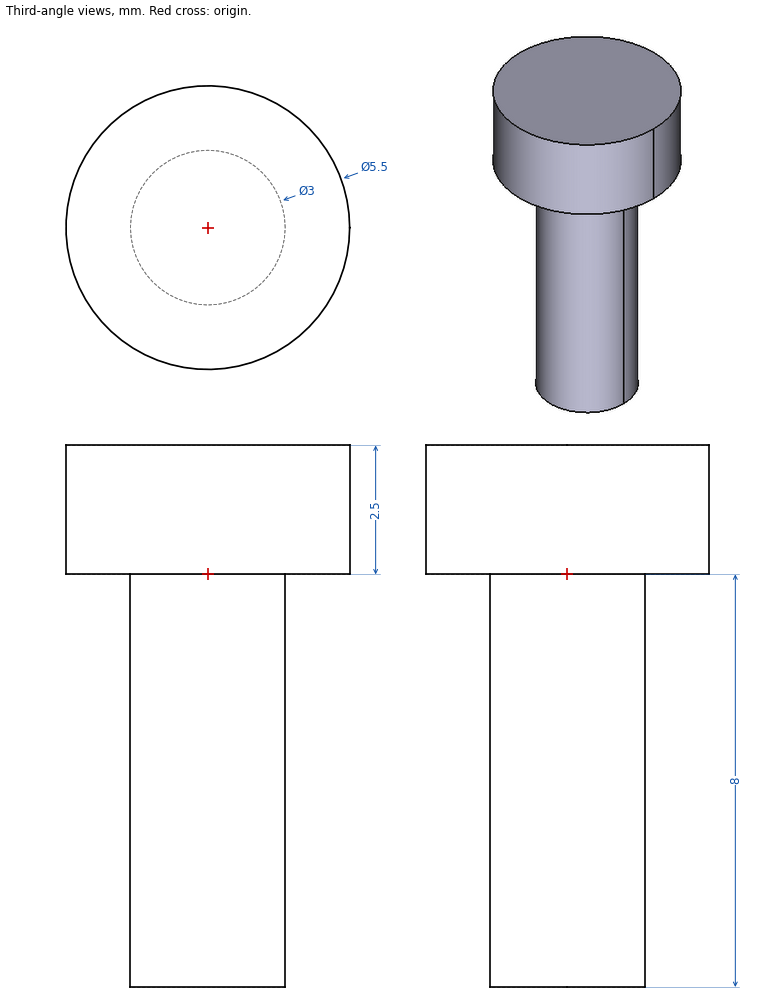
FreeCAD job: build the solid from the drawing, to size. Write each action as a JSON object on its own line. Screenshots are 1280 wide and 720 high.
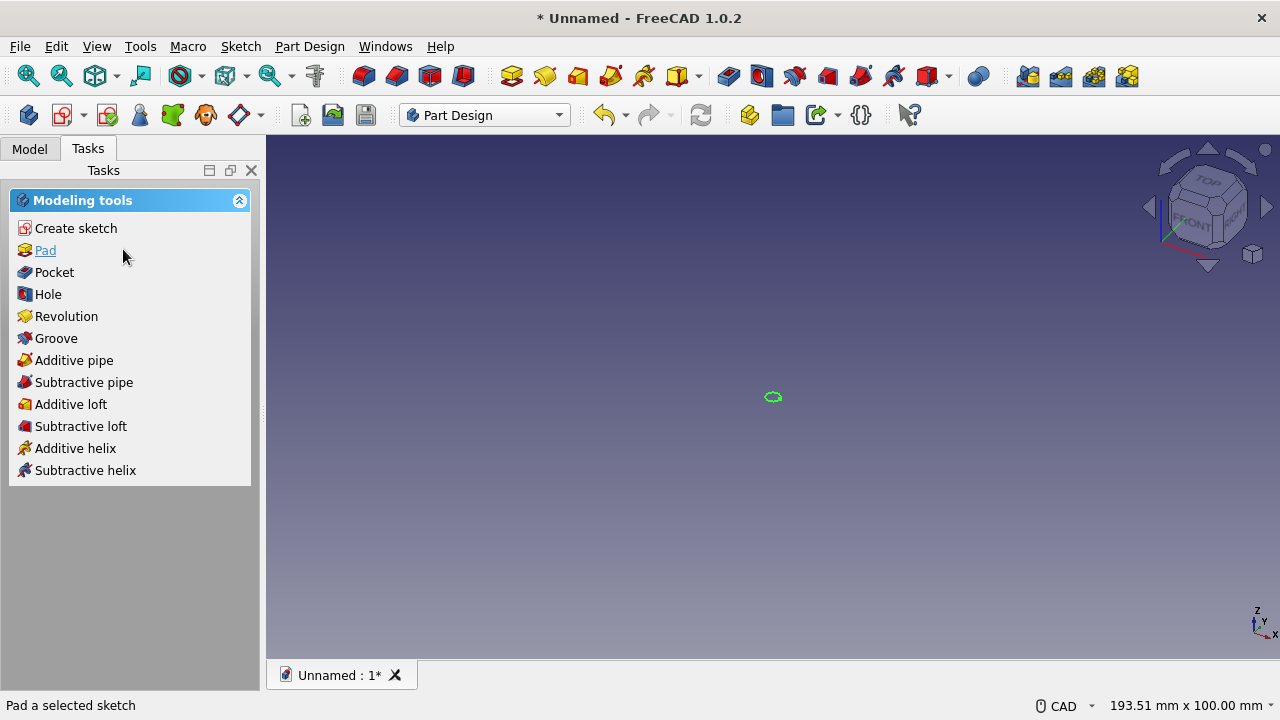
{"action": "left_click", "coordinate": [512, 76]}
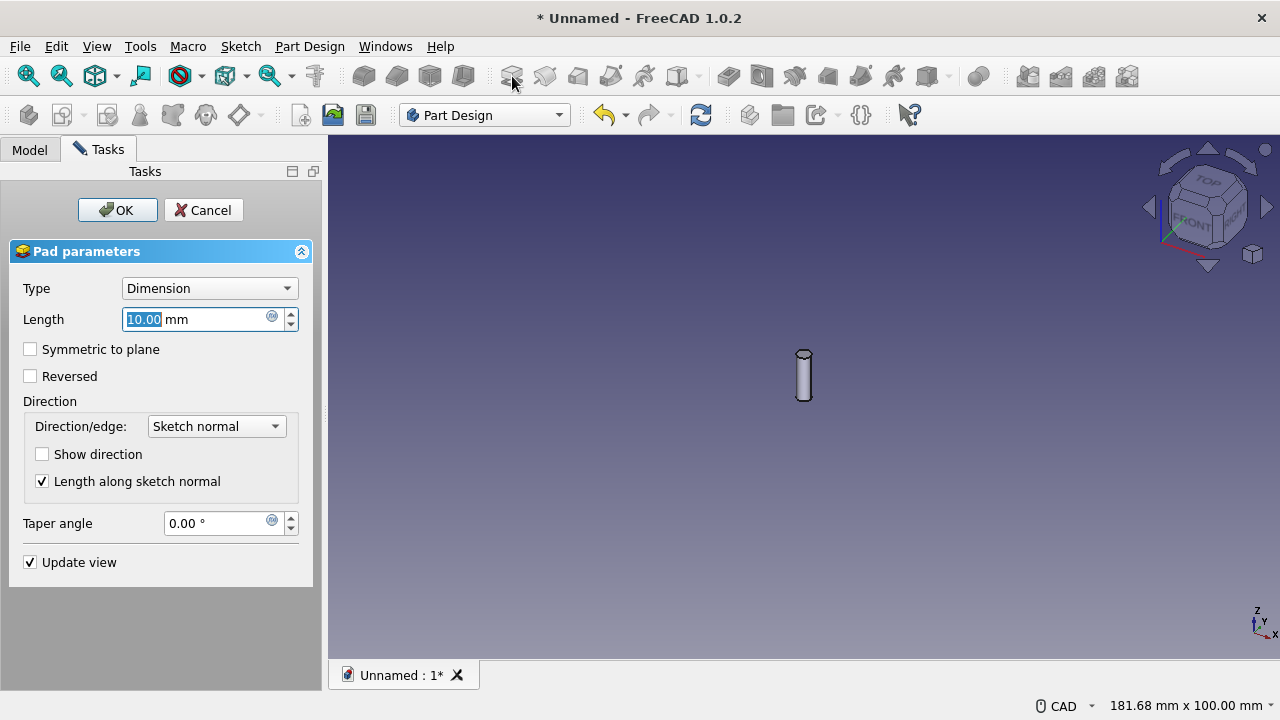
{"action": "type", "text": "8"}
{"action": "key", "text": "Tab"}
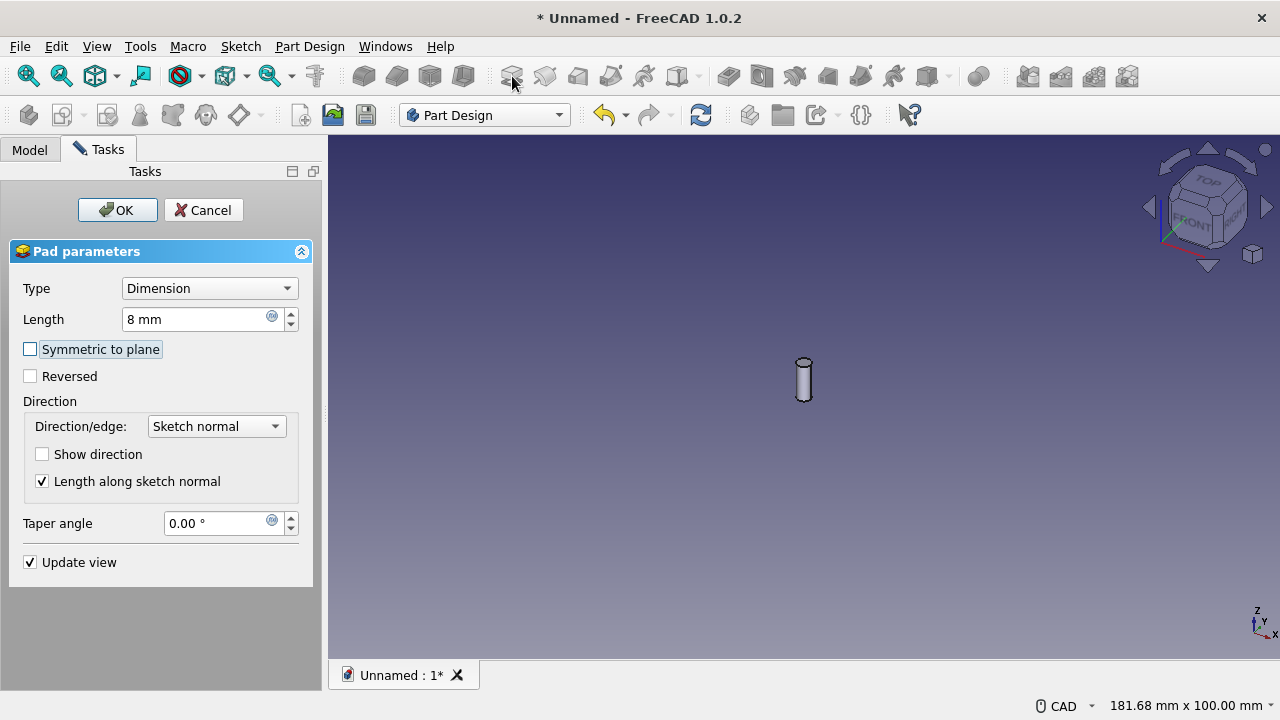
{"action": "left_click", "coordinate": [31, 376]}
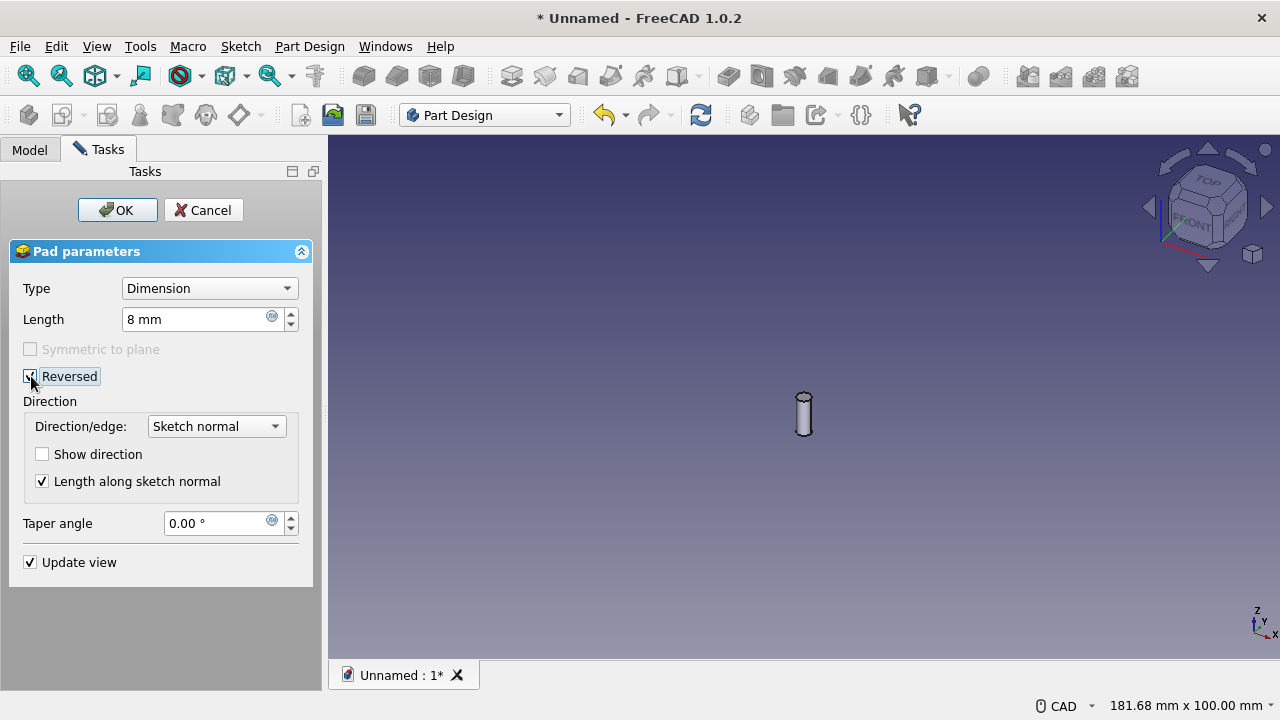
{"action": "left_click", "coordinate": [118, 210]}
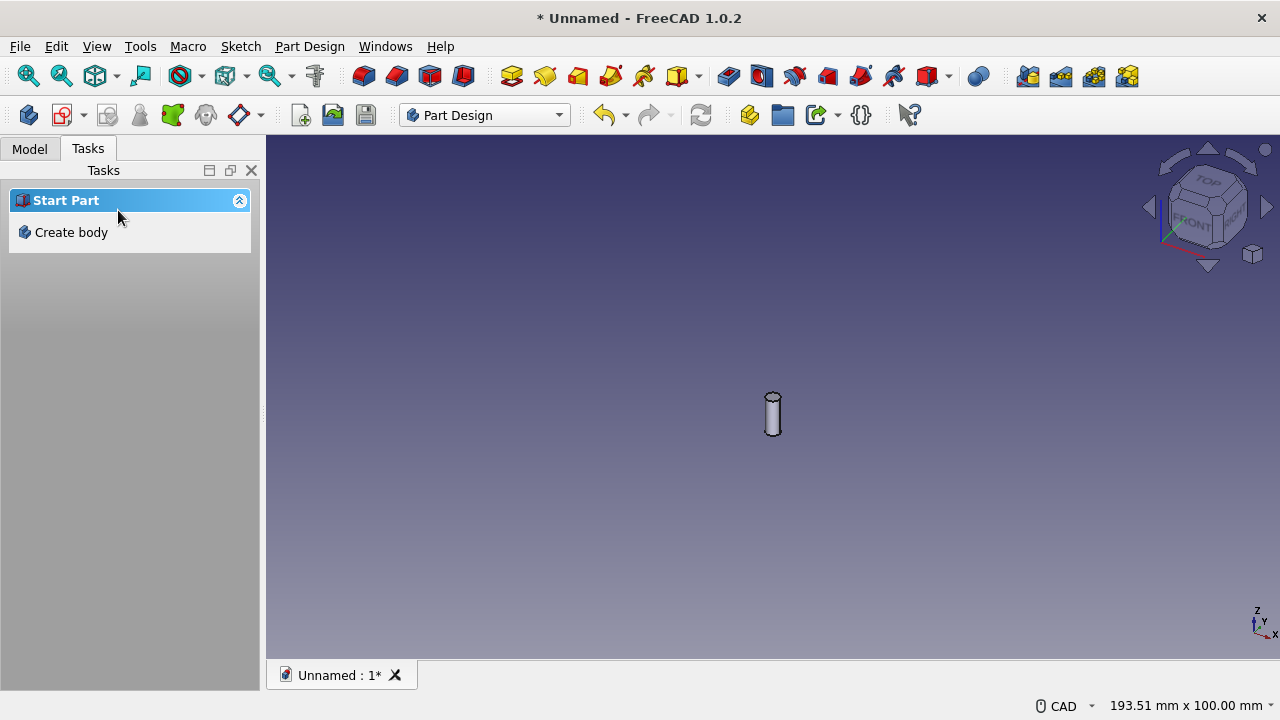
{"action": "left_click", "coordinate": [29, 76]}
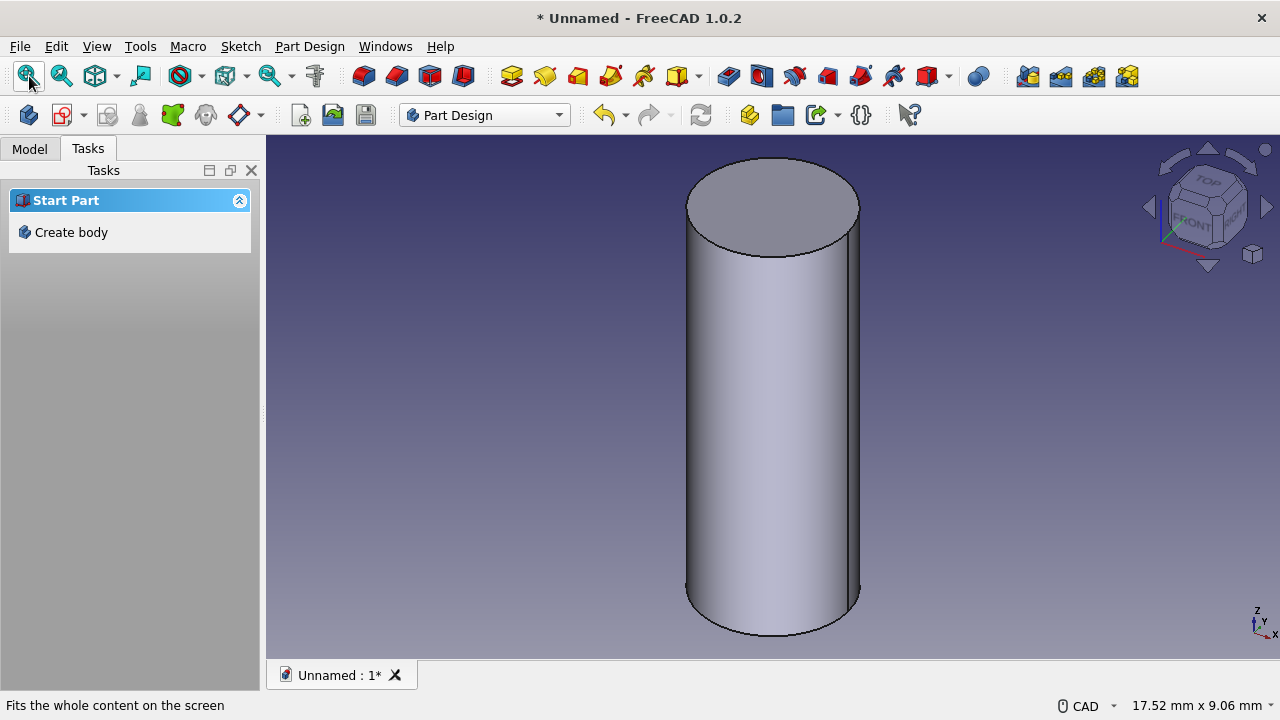
{"action": "left_click", "coordinate": [773, 206]}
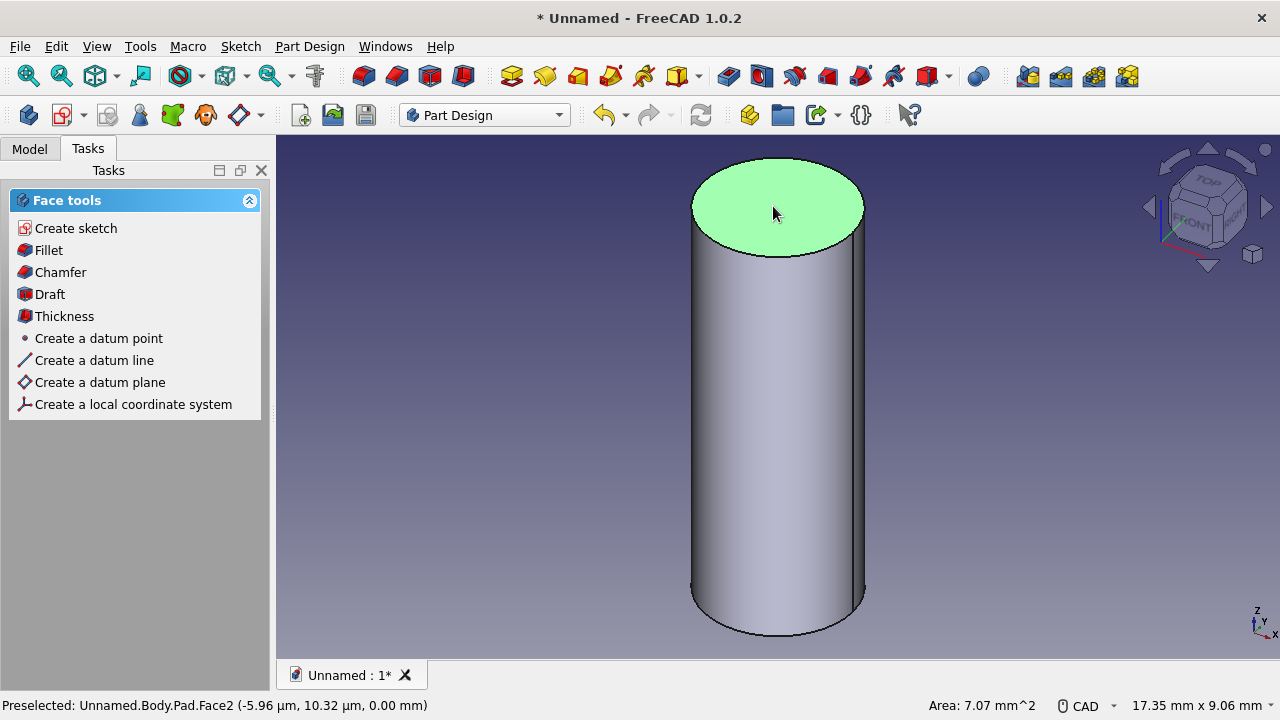
{"action": "left_click", "coordinate": [62, 116]}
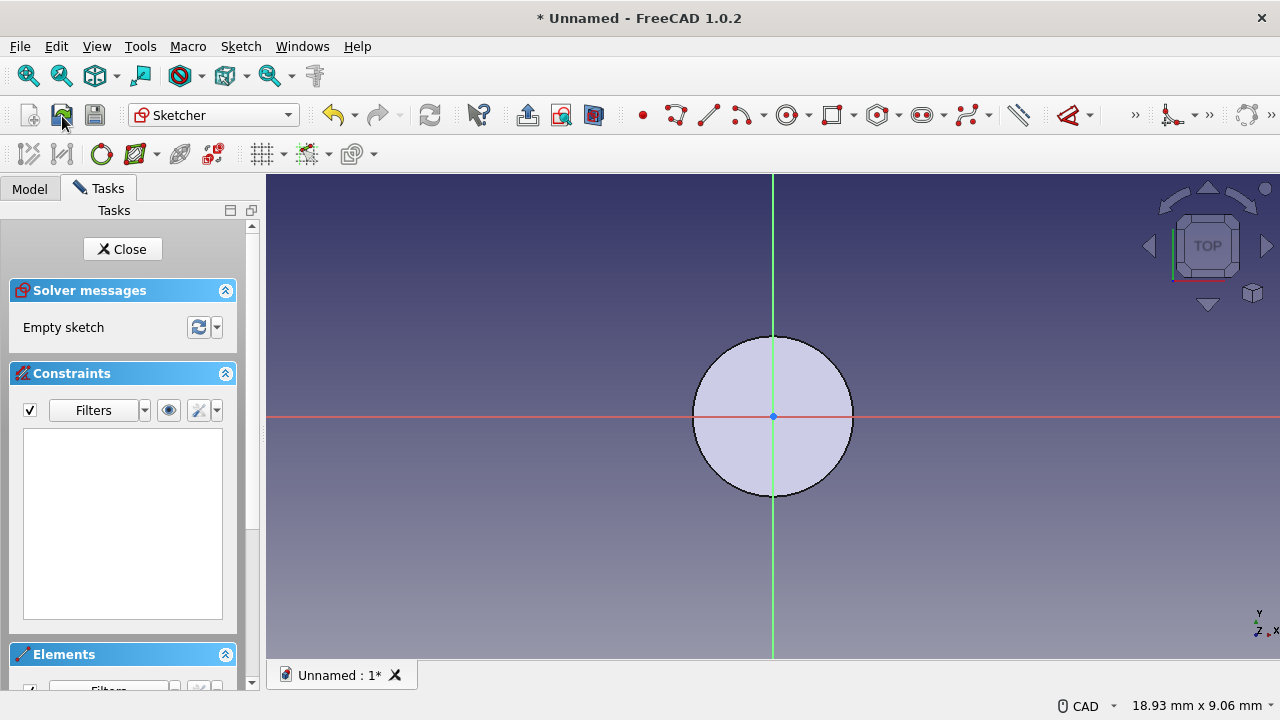
{"action": "left_click", "coordinate": [786, 116]}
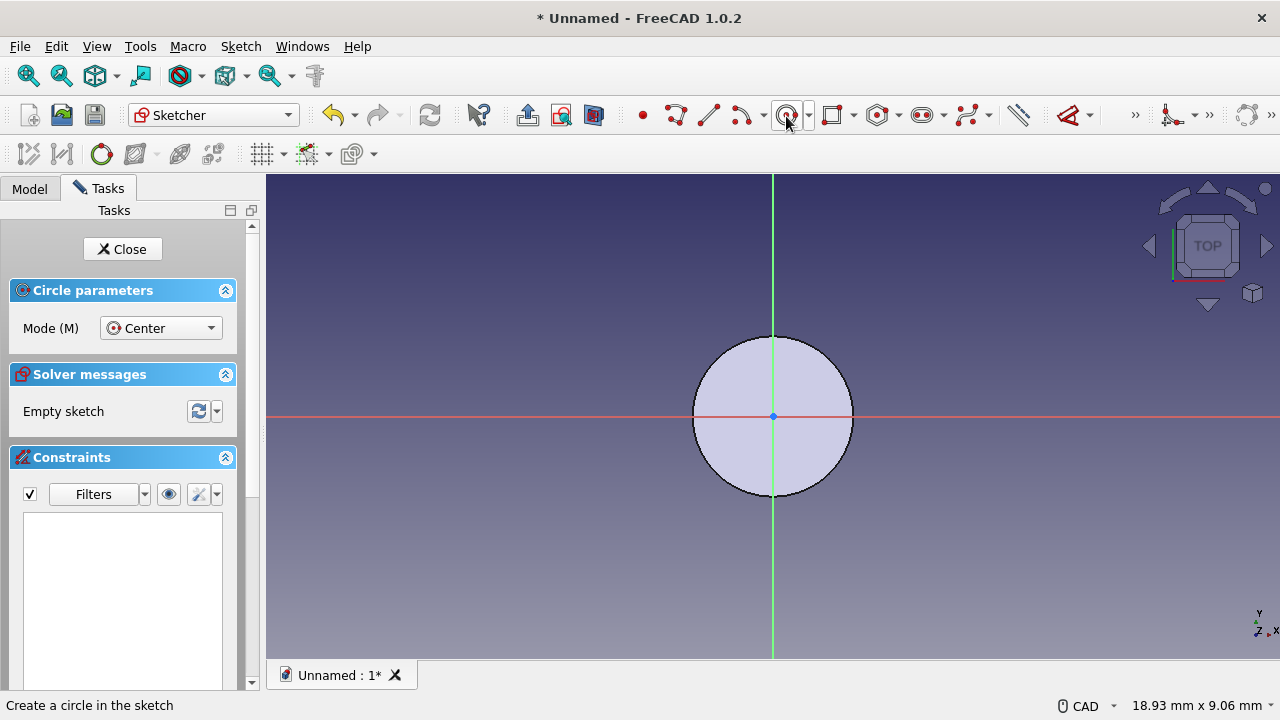
{"action": "left_click", "coordinate": [773, 416]}
{"action": "left_click", "coordinate": [877, 312]}
{"action": "key", "text": "Escape"}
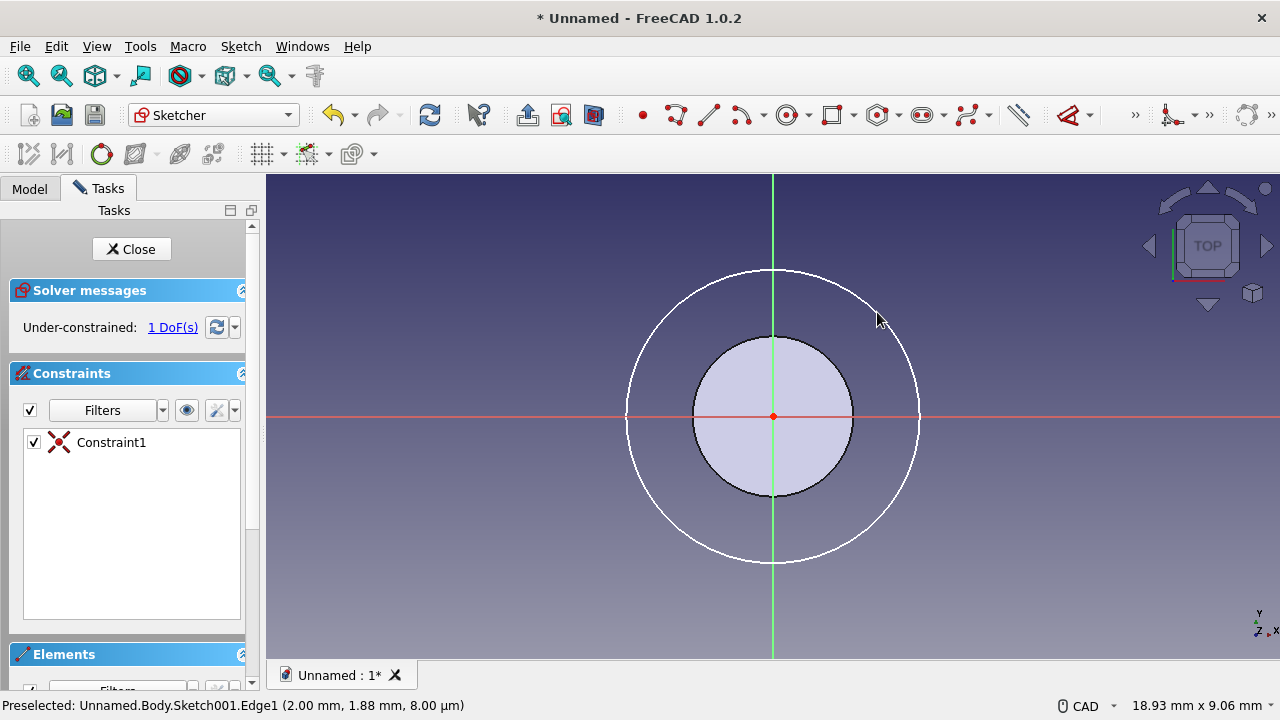
{"action": "left_click", "coordinate": [876, 312]}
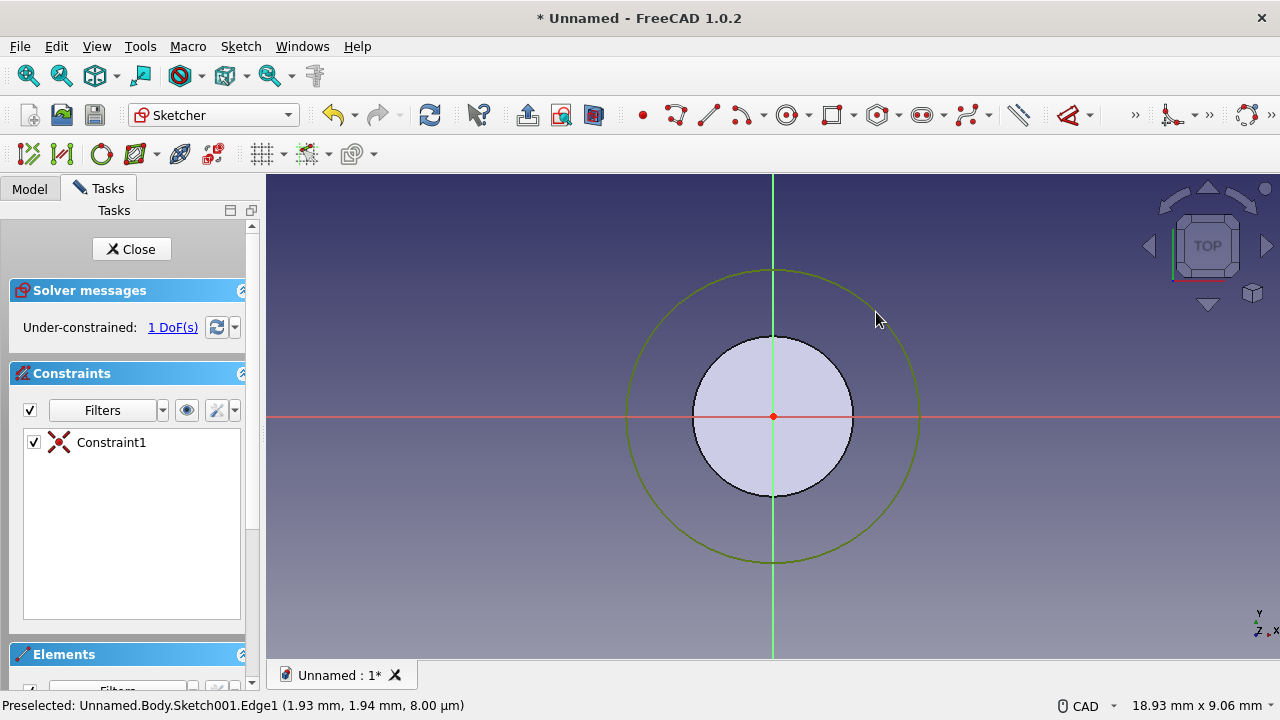
{"action": "left_click", "coordinate": [1090, 116]}